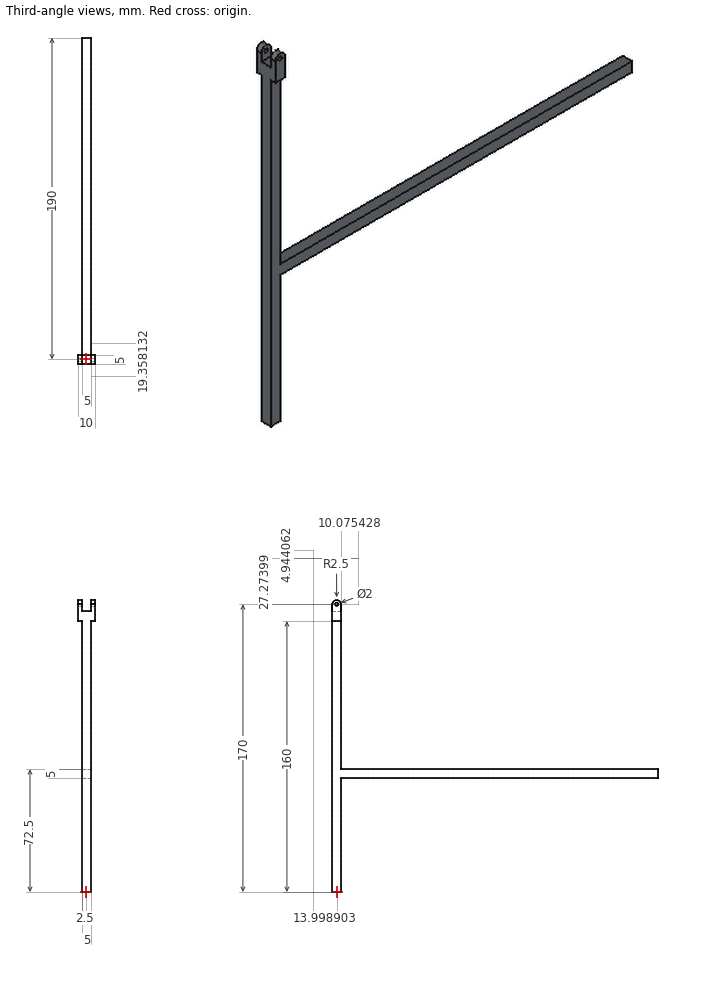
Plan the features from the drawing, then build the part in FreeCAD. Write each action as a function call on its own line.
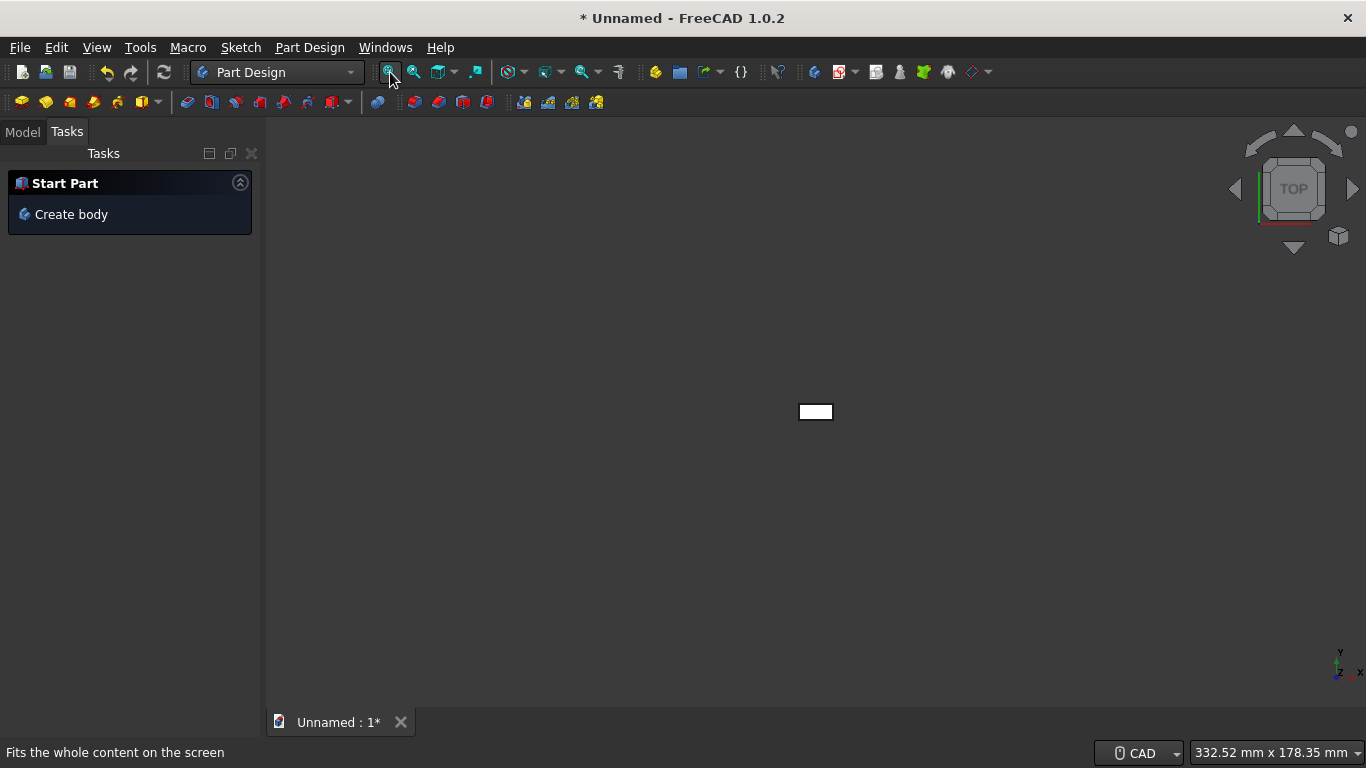
click(821, 411)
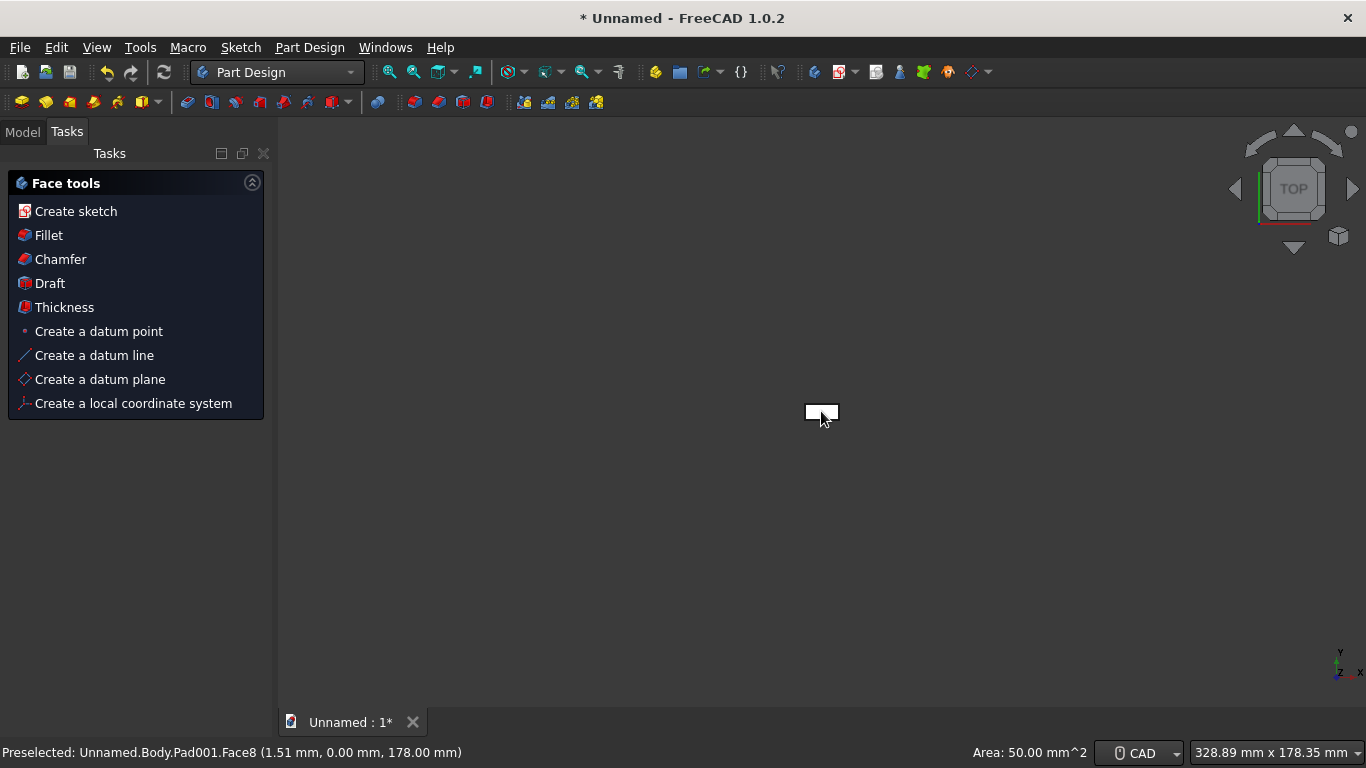
click(840, 72)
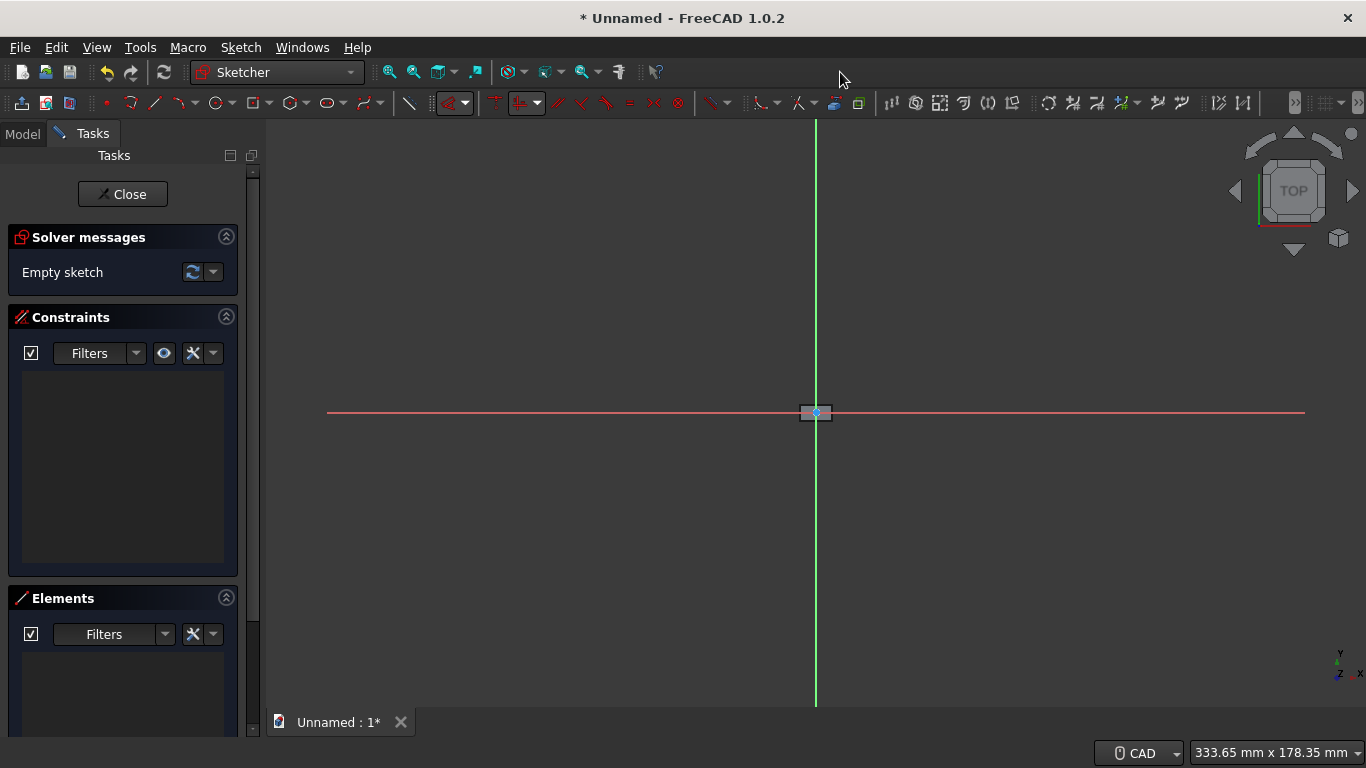
scroll(830, 413, up, 9)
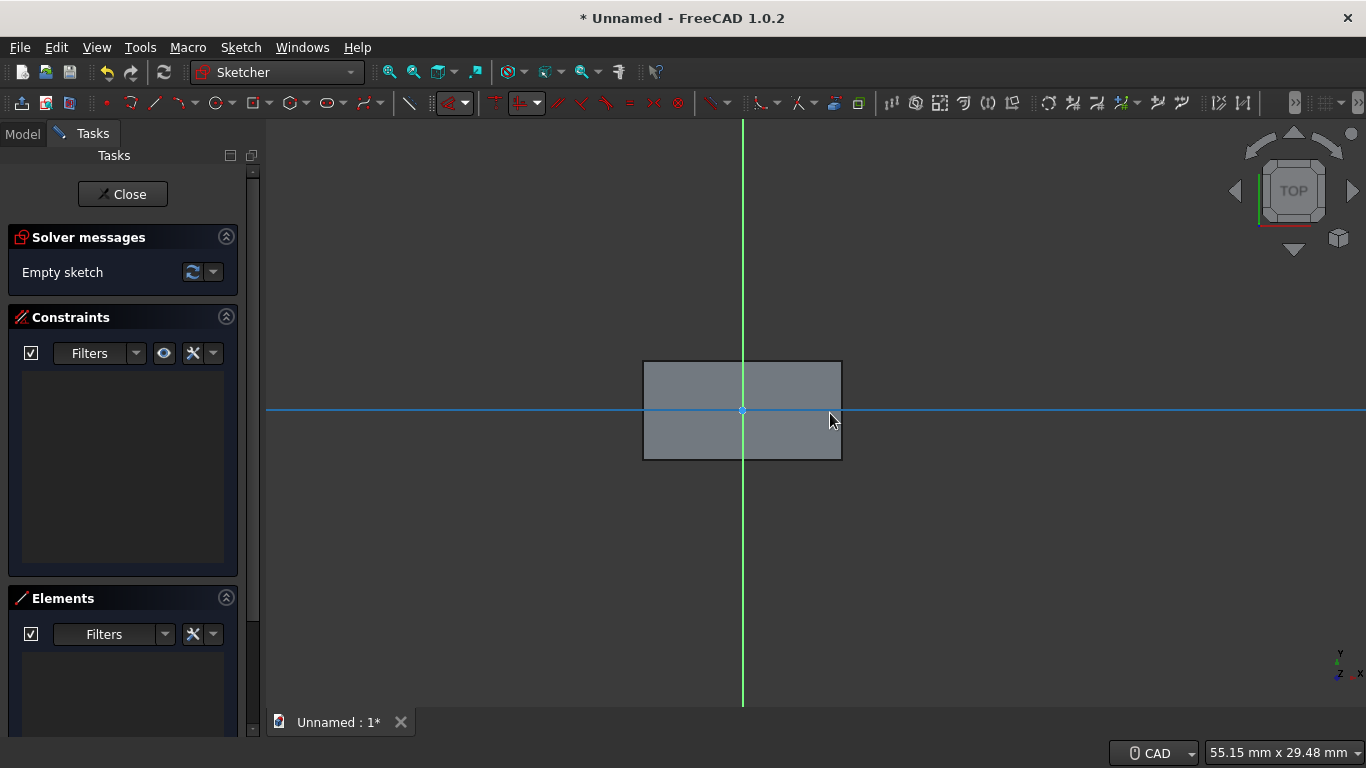
click(254, 104)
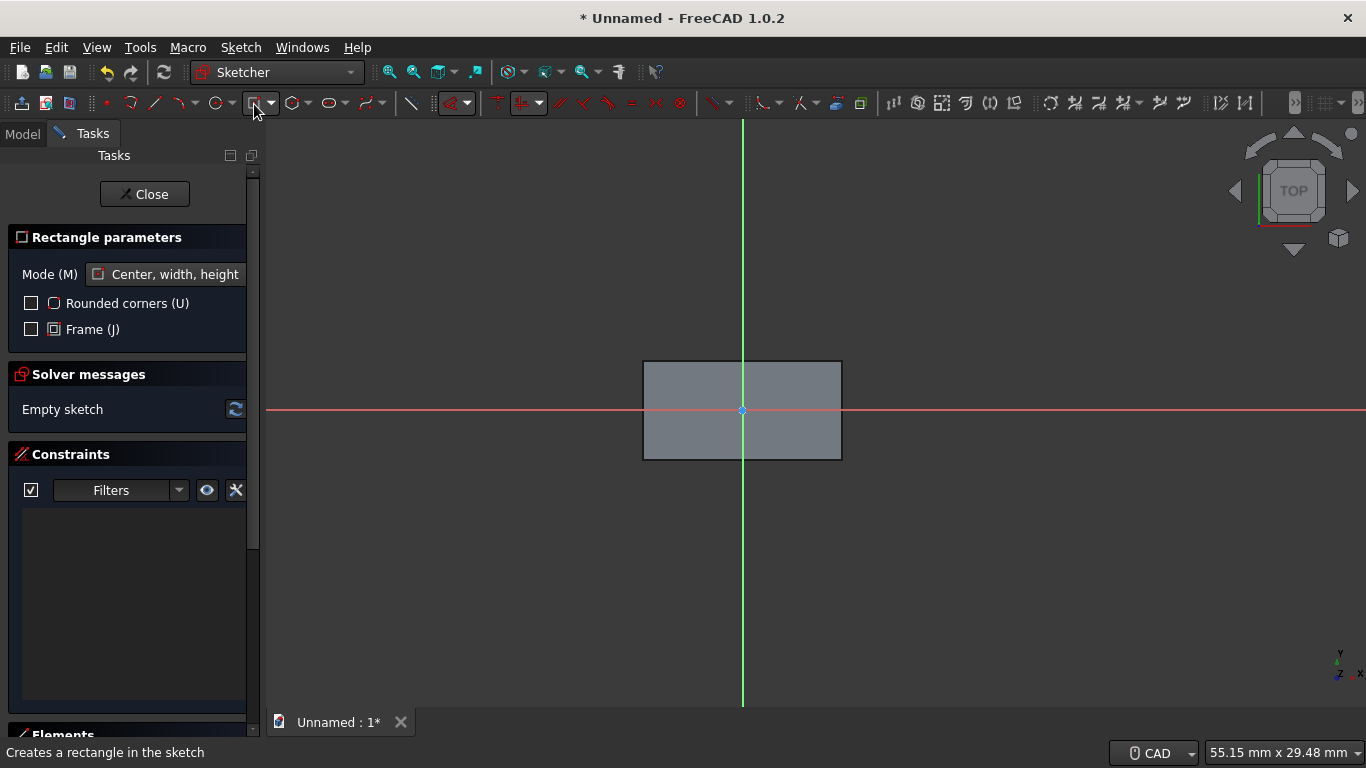
click(743, 410)
click(793, 217)
key(Escape)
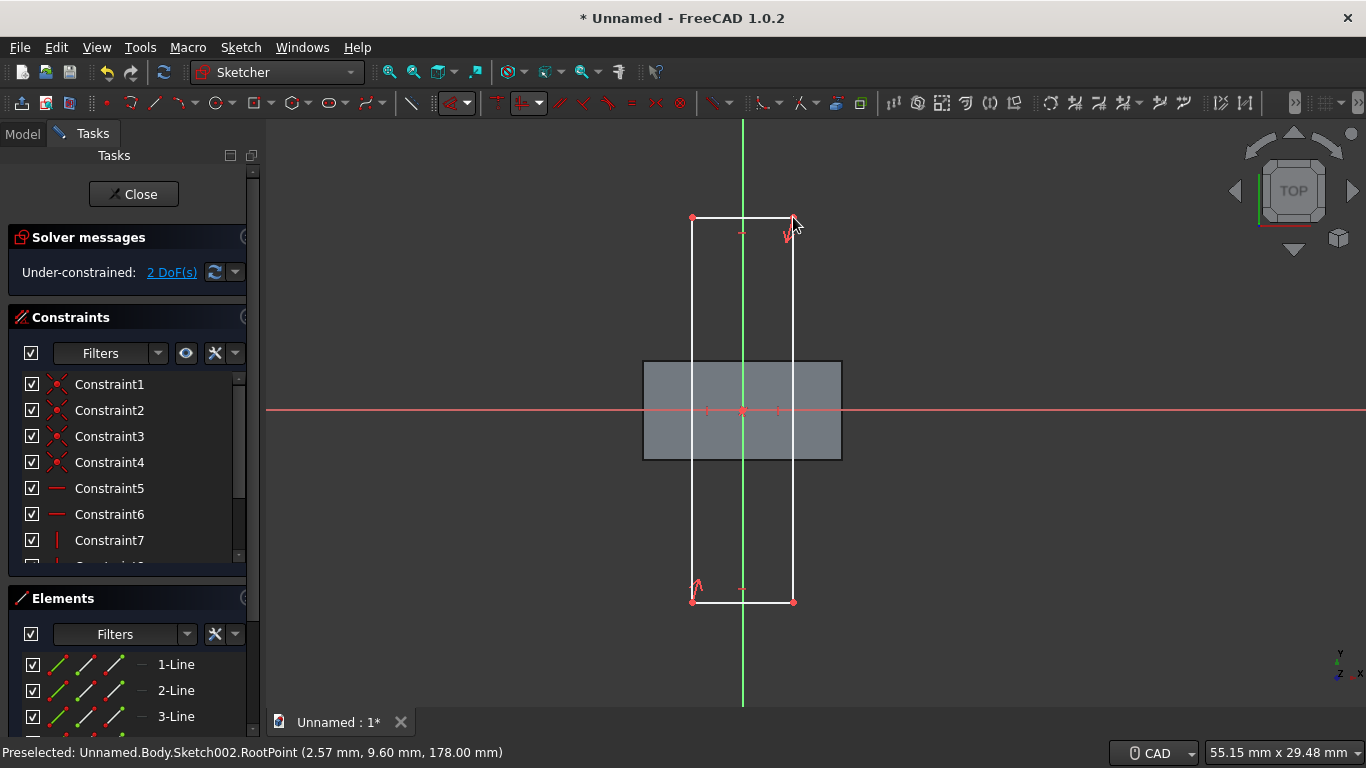
click(723, 603)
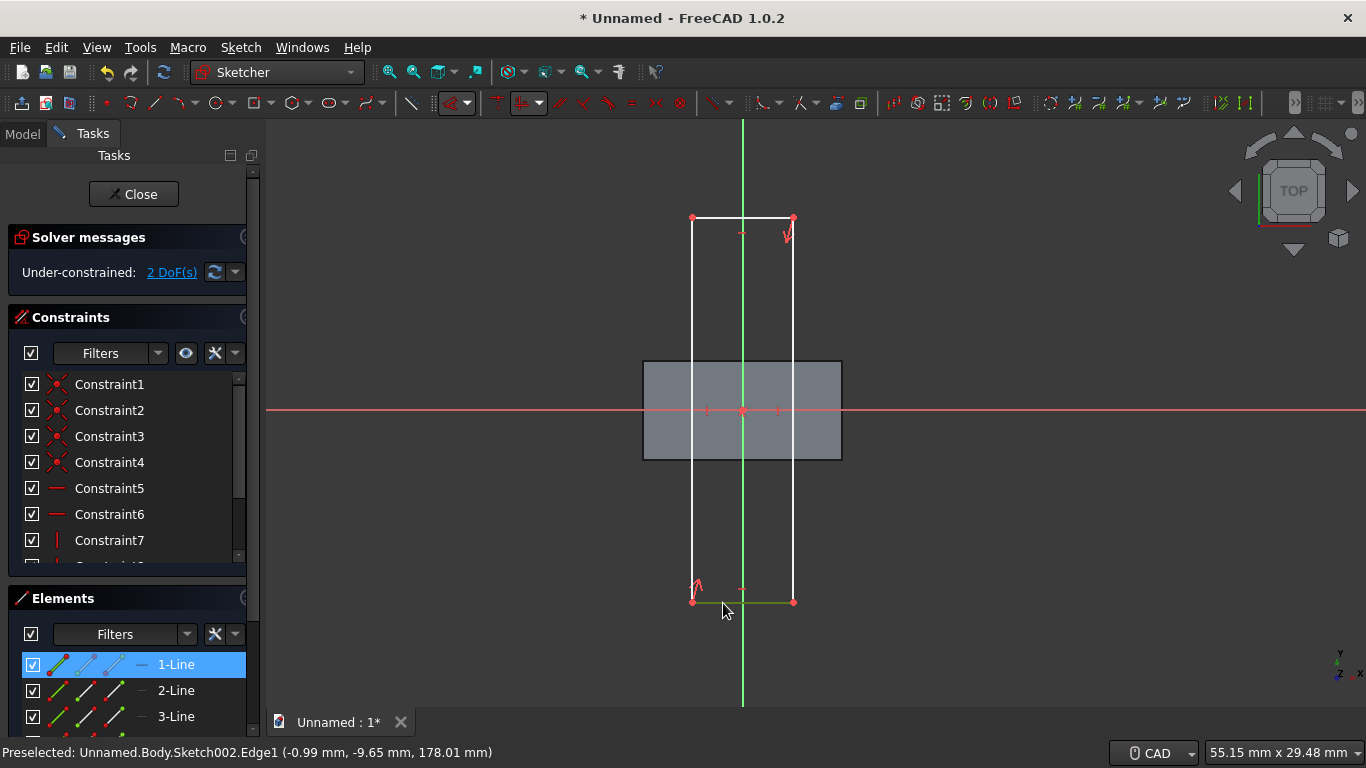
click(470, 104)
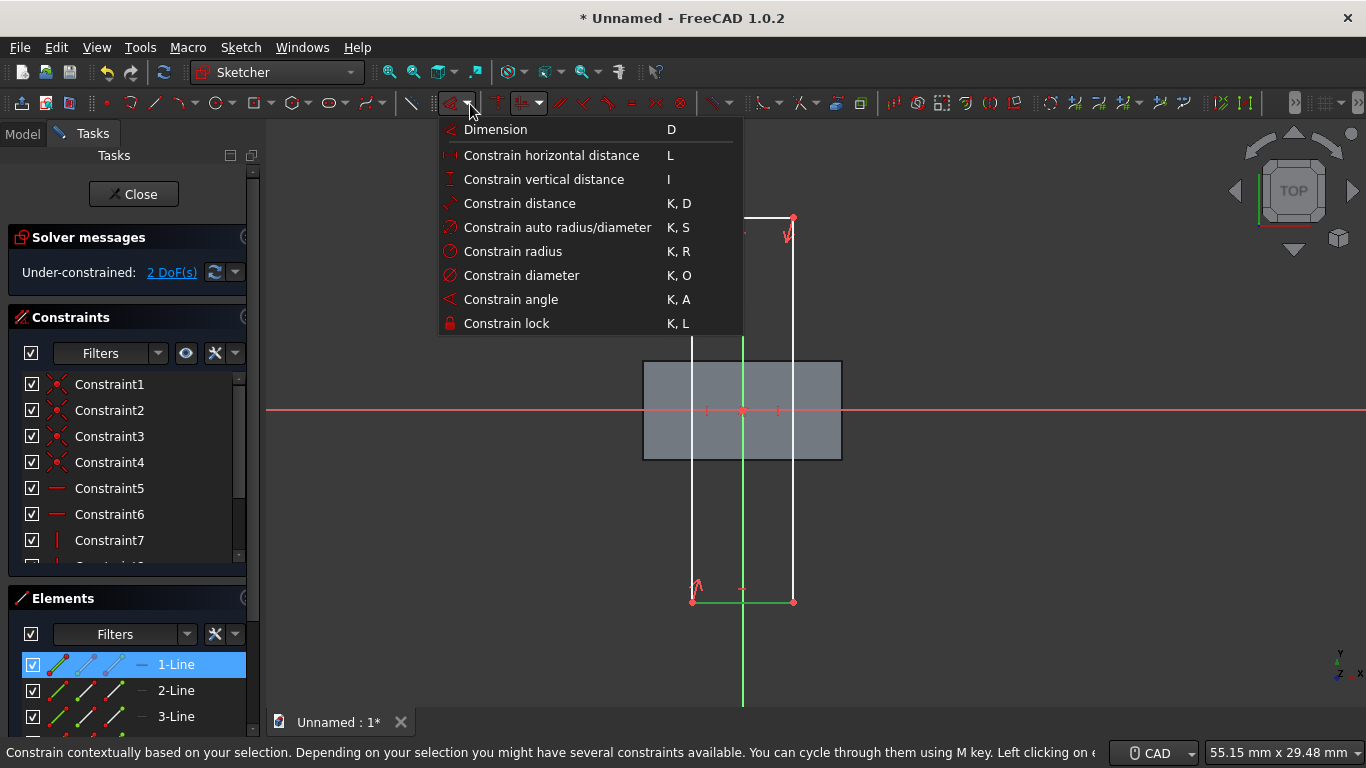
click(591, 155)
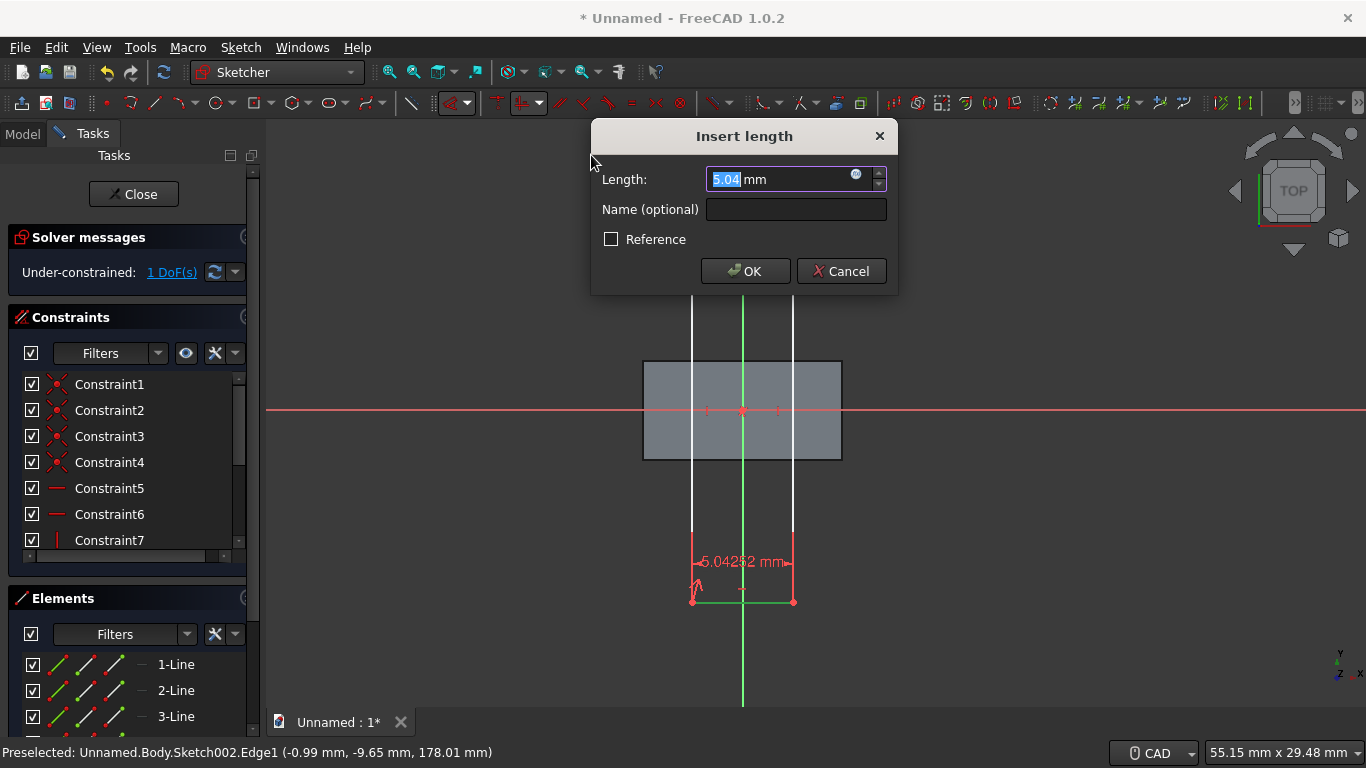
text(5)
key(Return)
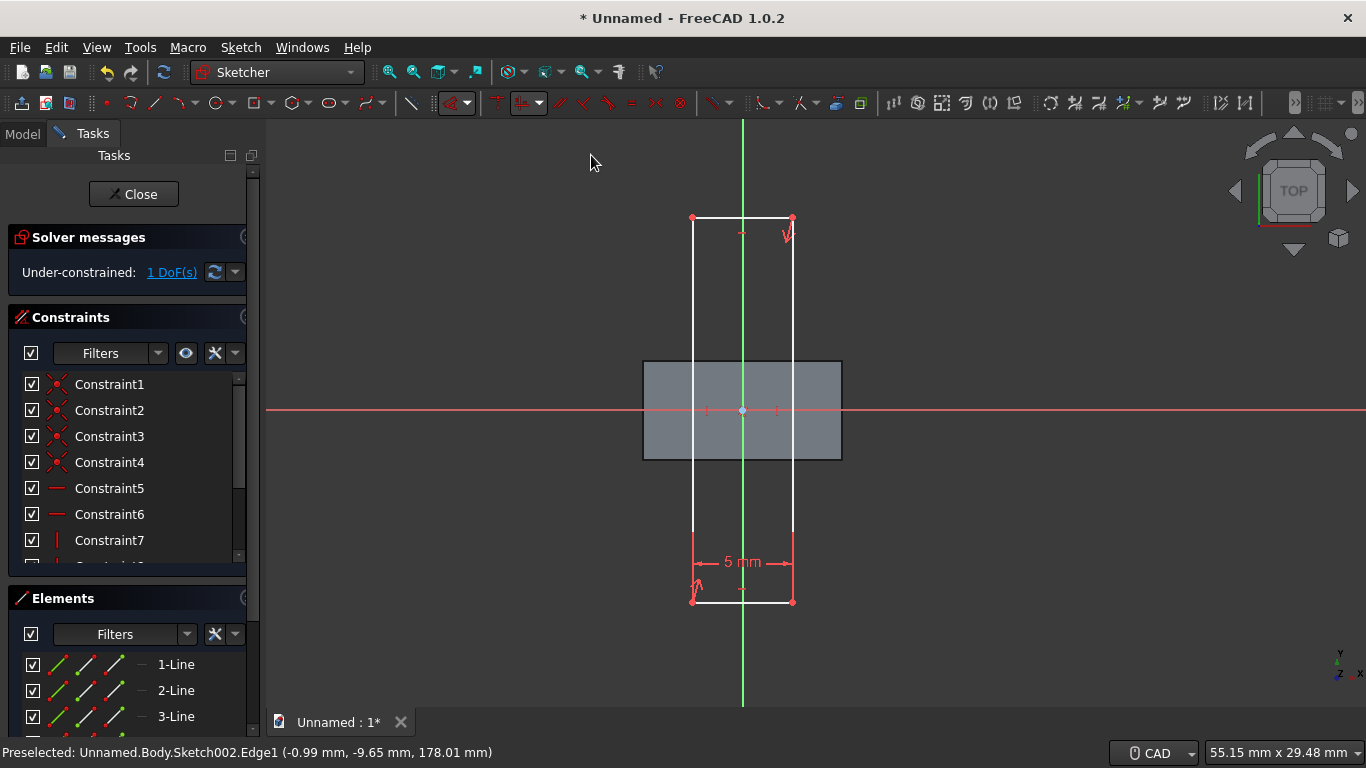
click(793, 487)